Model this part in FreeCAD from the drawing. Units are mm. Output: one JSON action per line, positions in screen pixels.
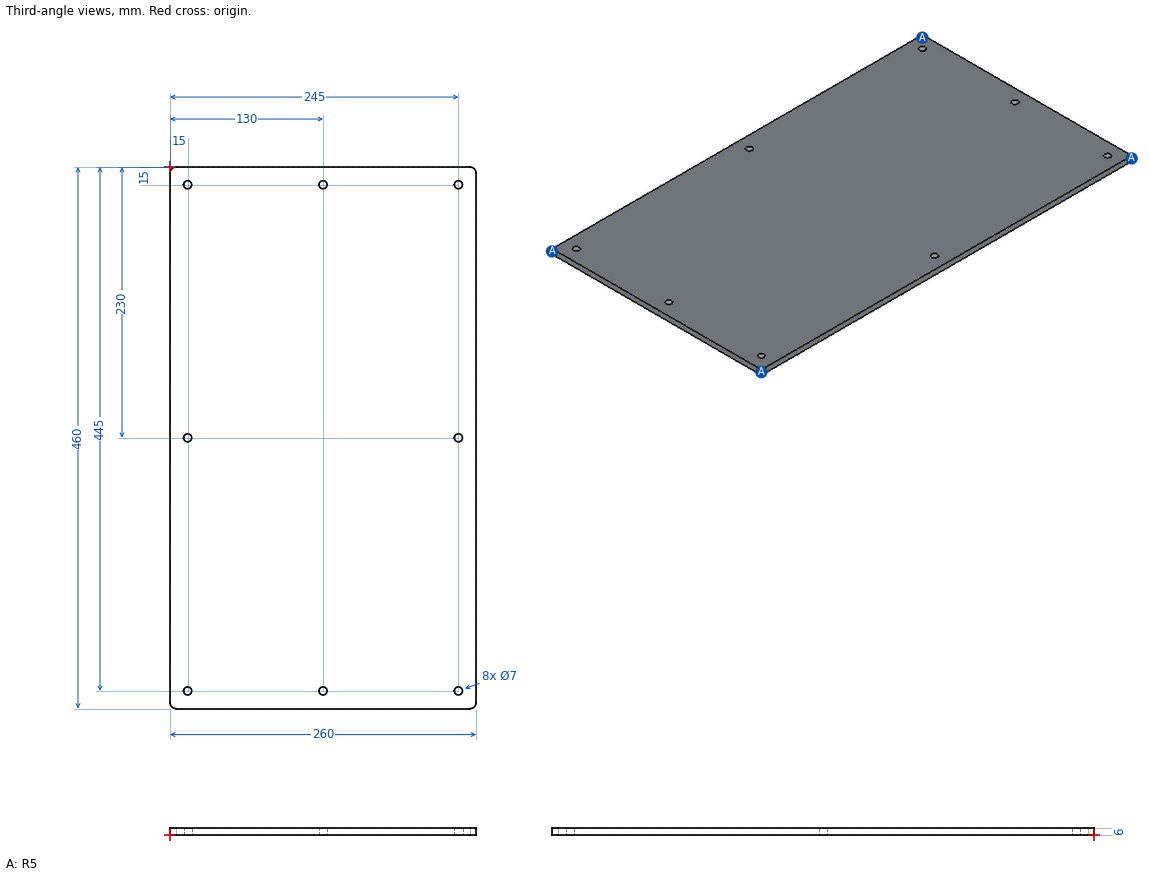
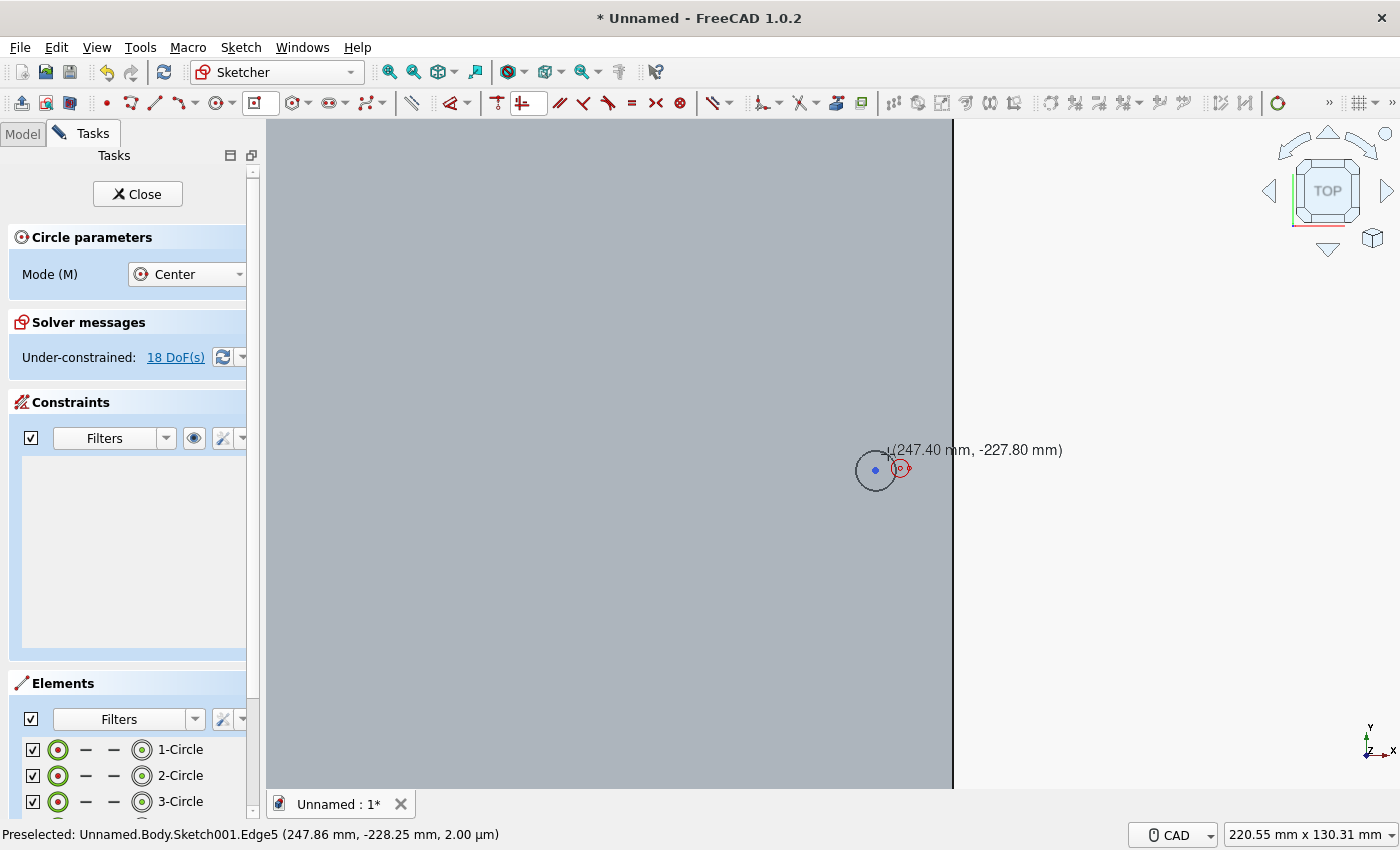
{"action": "scroll", "coordinate": [893, 458], "scroll_direction": "down", "scroll_amount": 8}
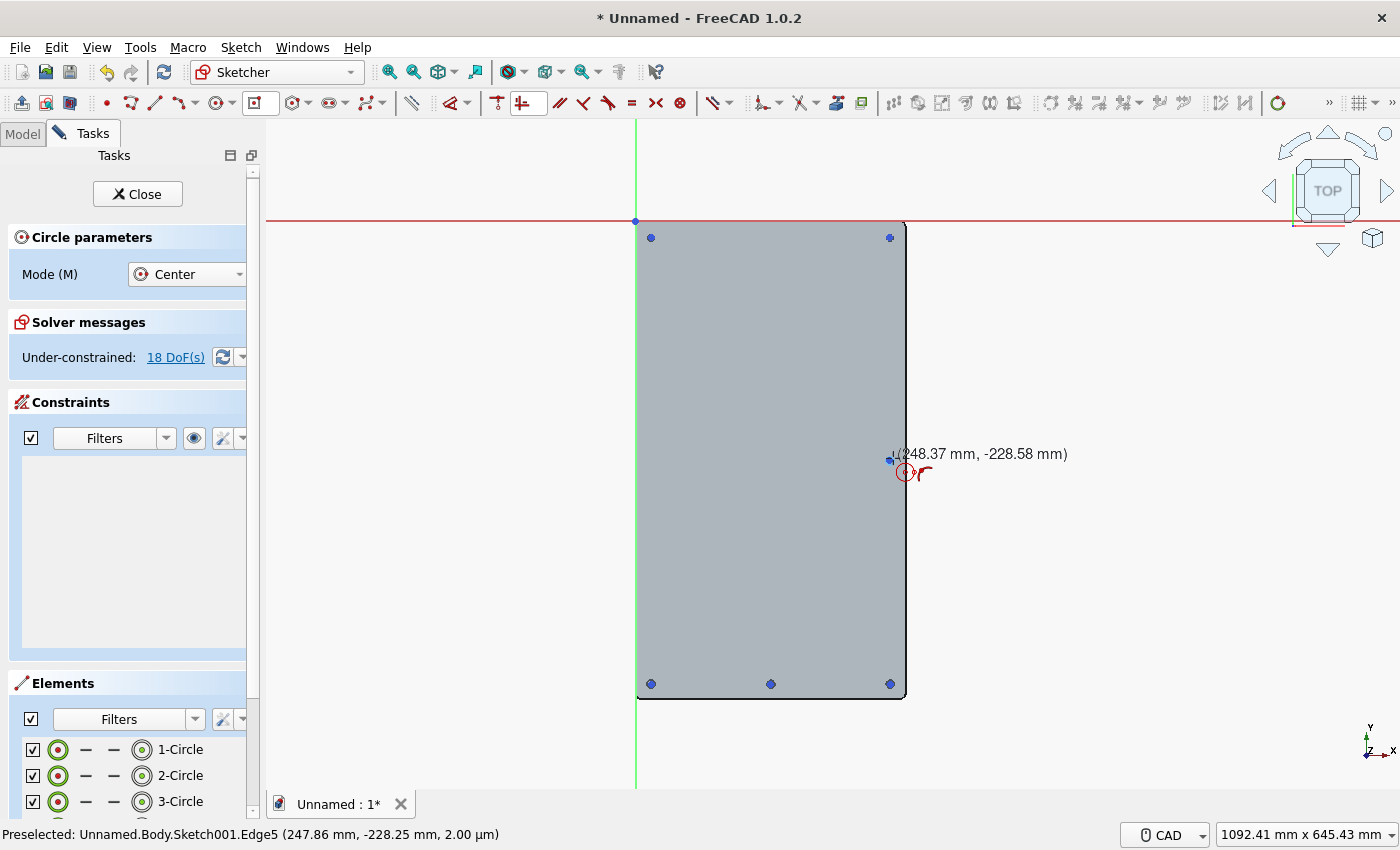
{"action": "scroll", "coordinate": [771, 237], "scroll_direction": "up", "scroll_amount": 10}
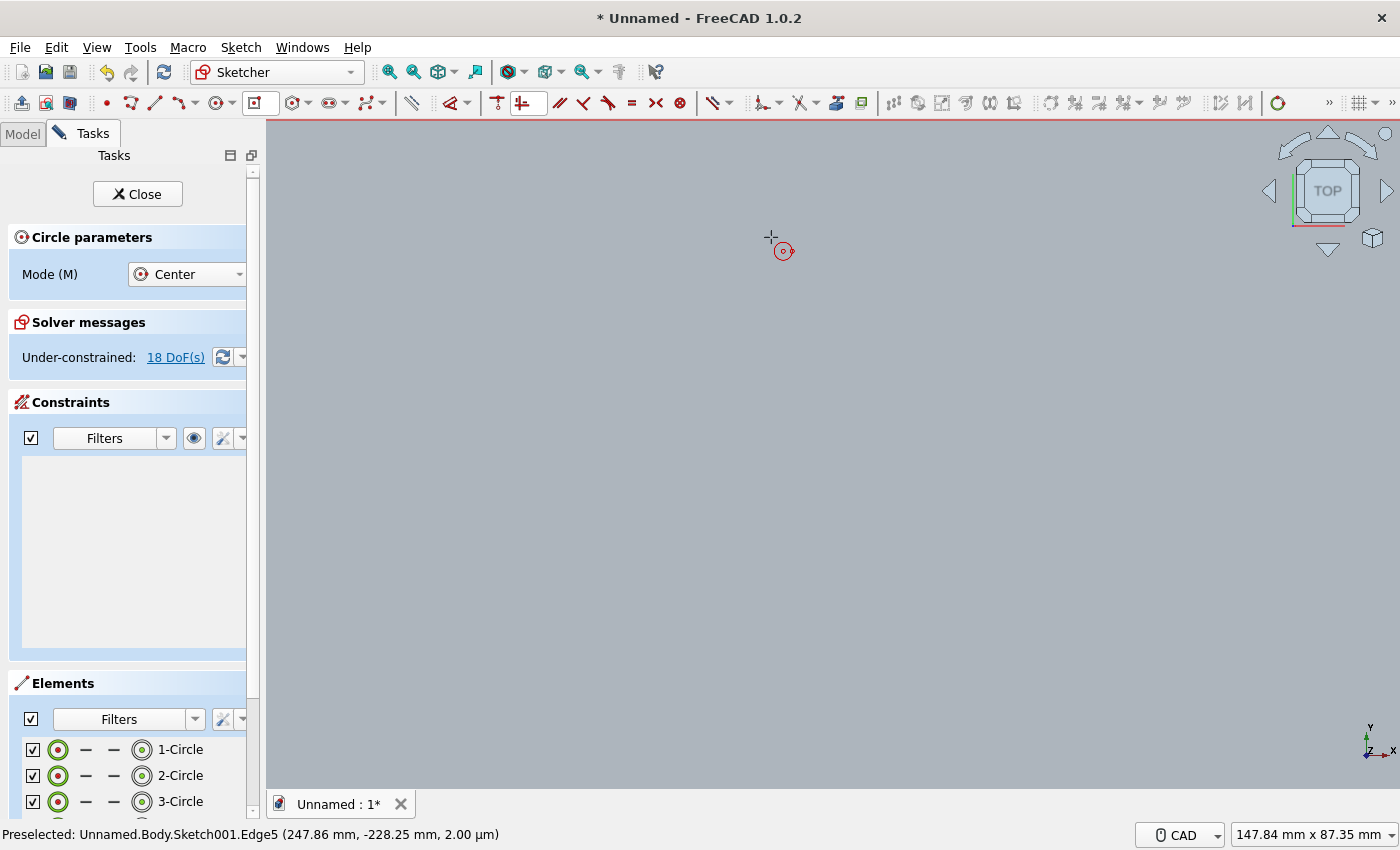
{"action": "scroll", "coordinate": [771, 237], "scroll_direction": "down", "scroll_amount": 10}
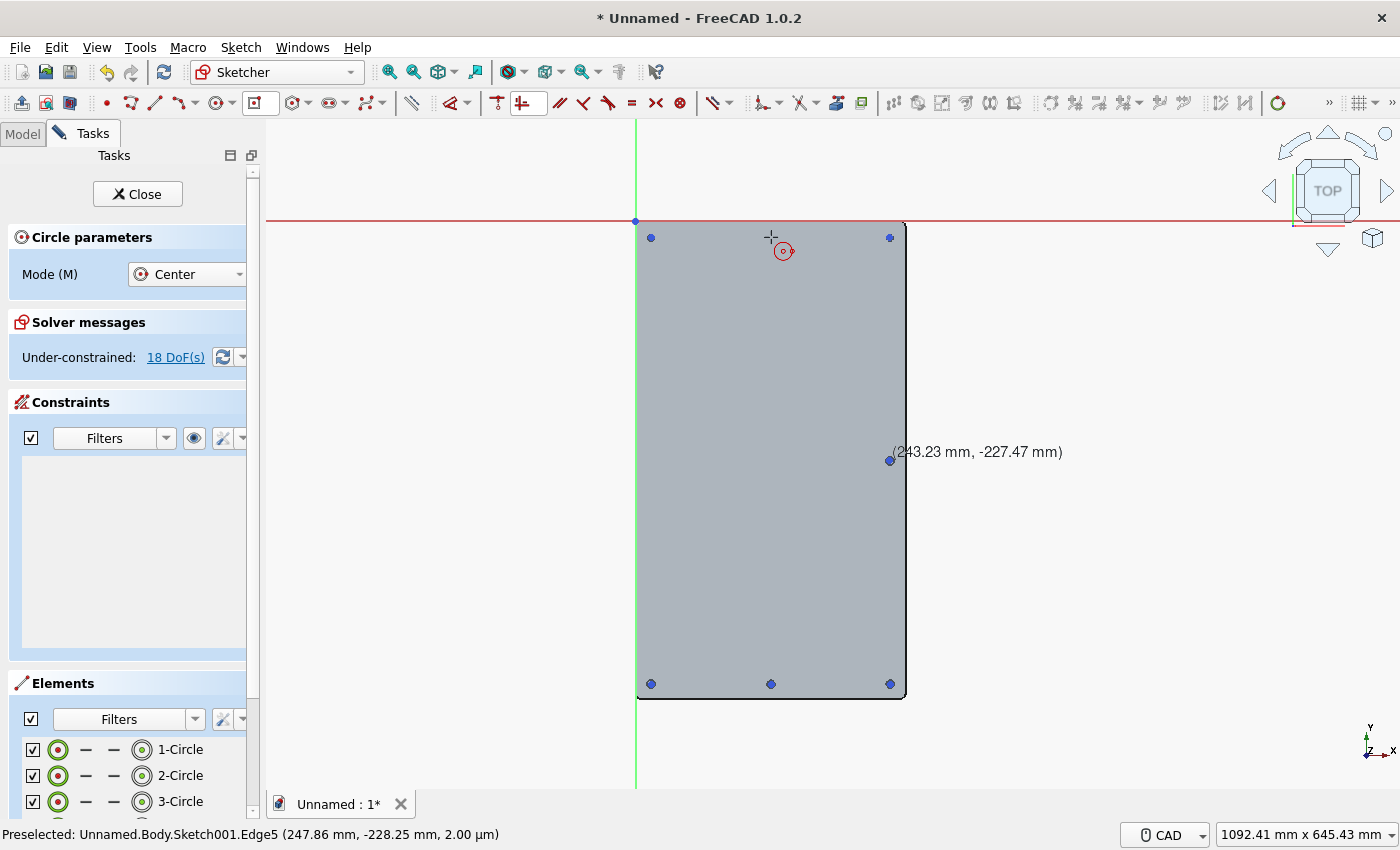
{"action": "left_click", "coordinate": [771, 237]}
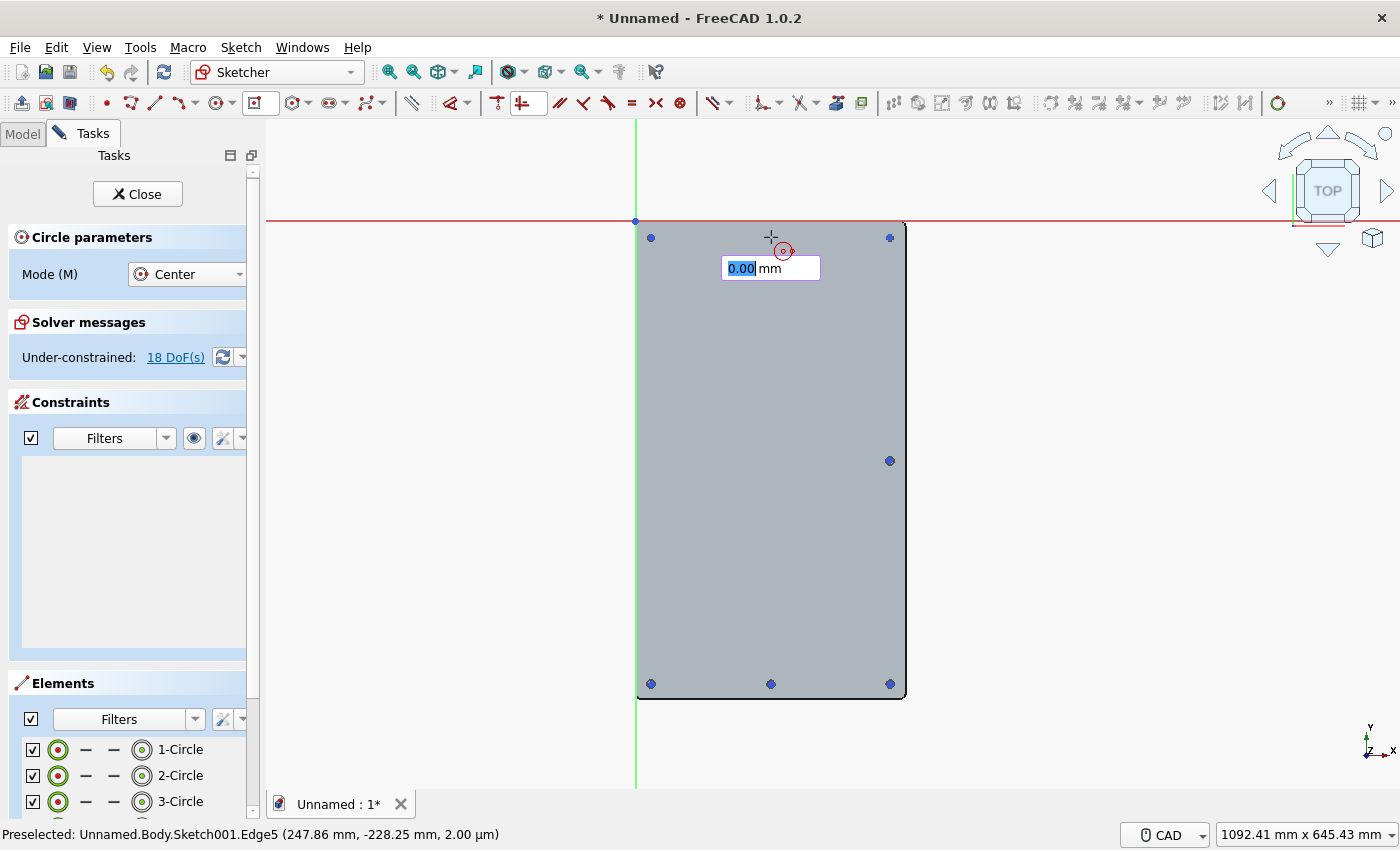
{"action": "scroll", "coordinate": [773, 239], "scroll_direction": "up", "scroll_amount": 8}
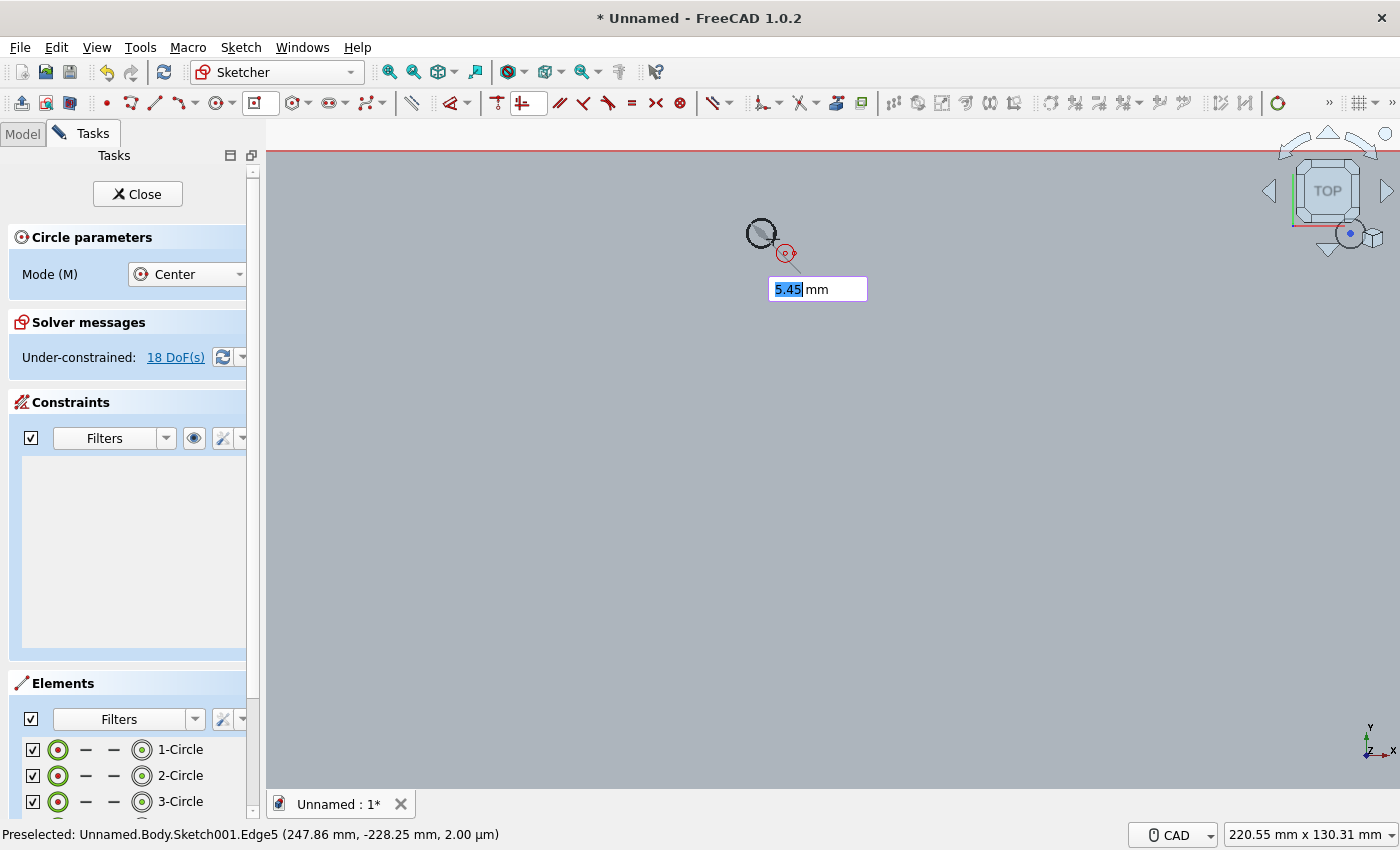
{"action": "left_click", "coordinate": [772, 241]}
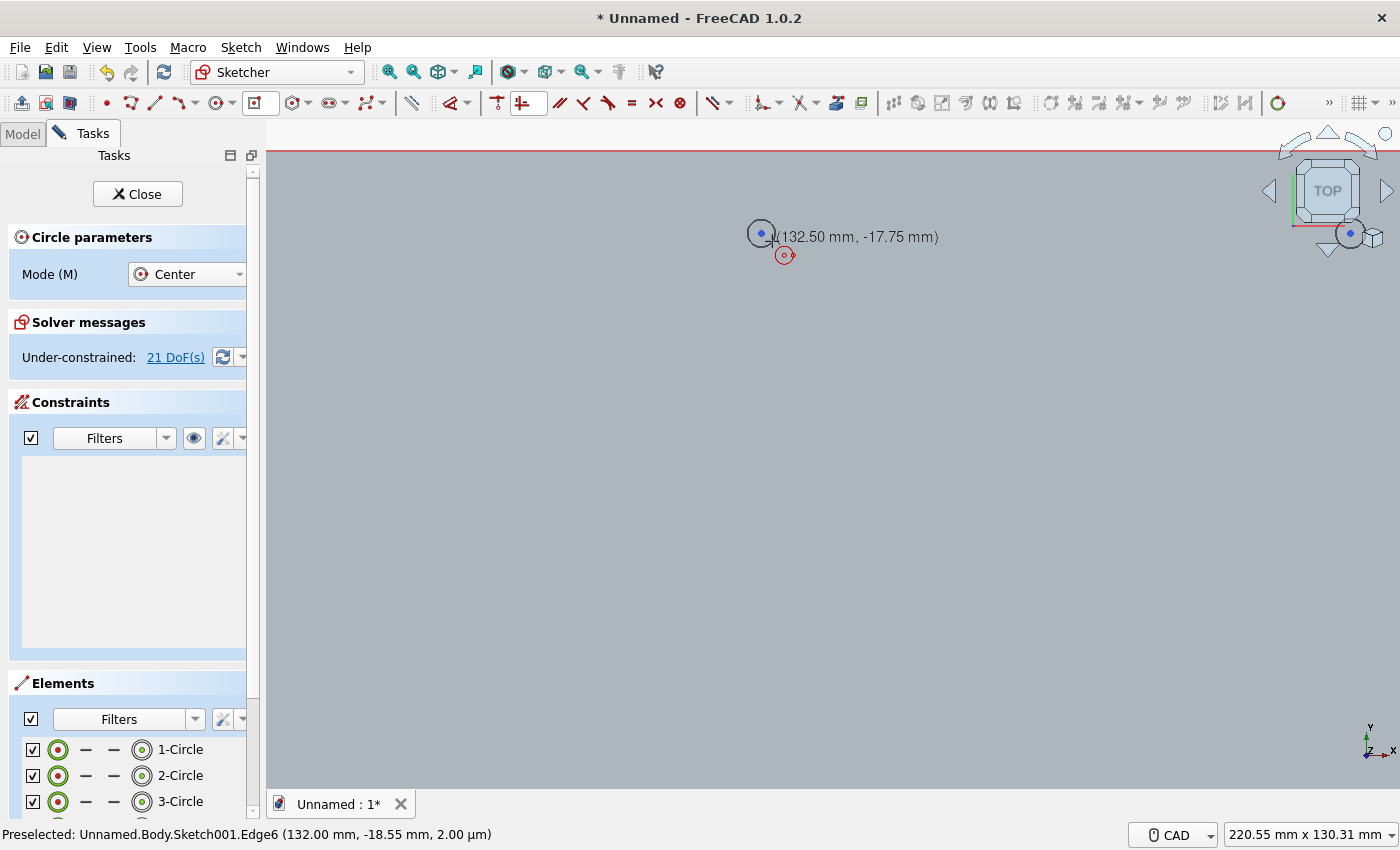
{"action": "scroll", "coordinate": [773, 239], "scroll_direction": "down", "scroll_amount": 8}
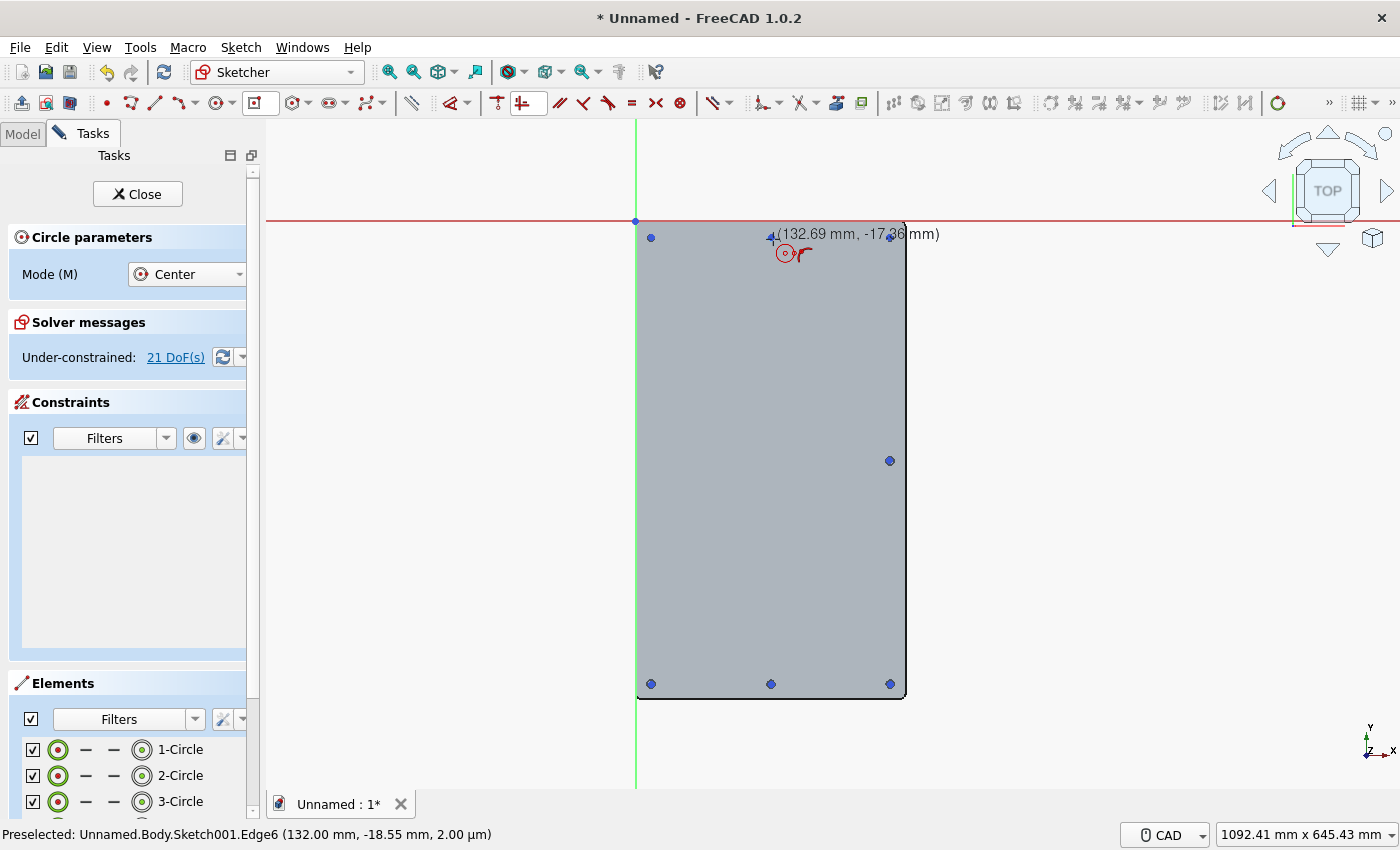
{"action": "scroll", "coordinate": [651, 460], "scroll_direction": "up", "scroll_amount": 10}